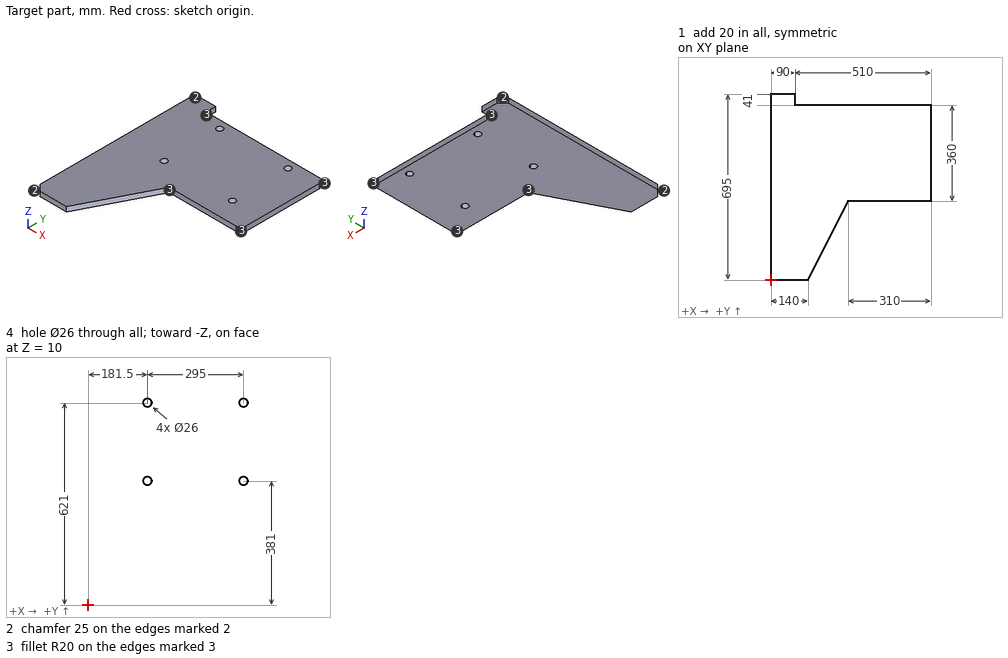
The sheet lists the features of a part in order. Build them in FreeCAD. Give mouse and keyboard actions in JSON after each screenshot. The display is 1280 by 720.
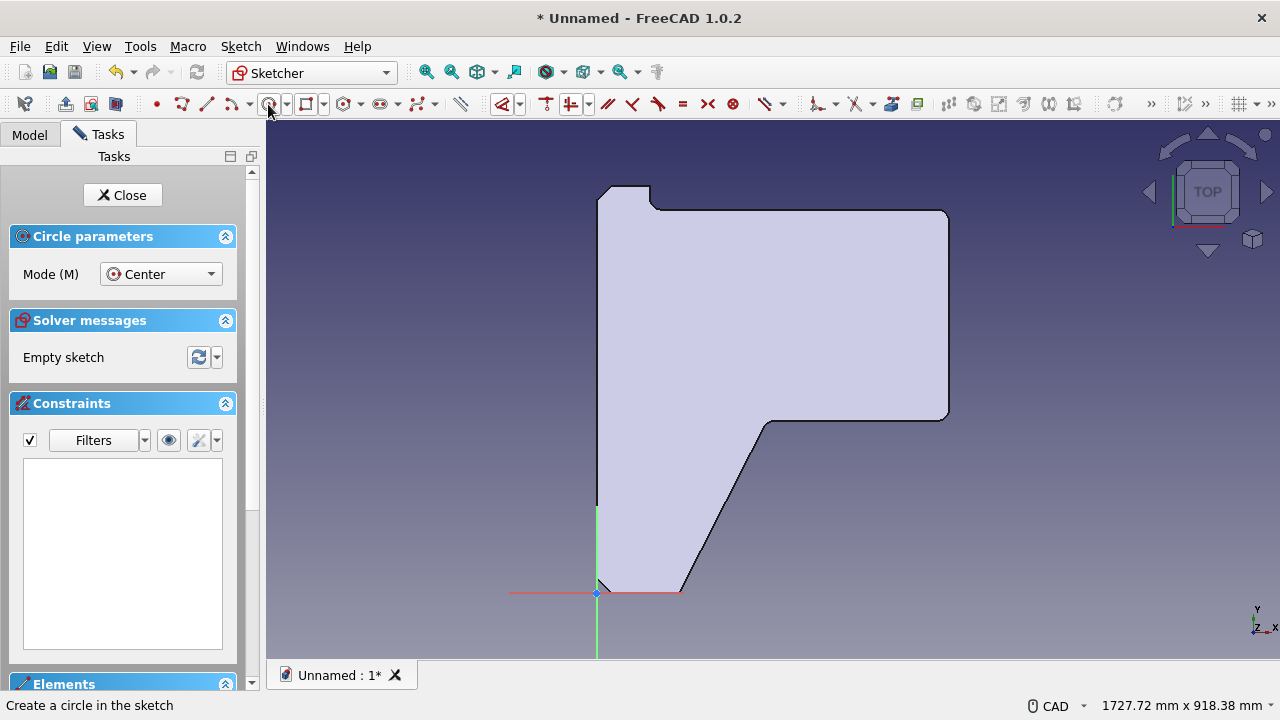
{"action": "scroll", "coordinate": [703, 229], "scroll_direction": "up", "scroll_amount": 6}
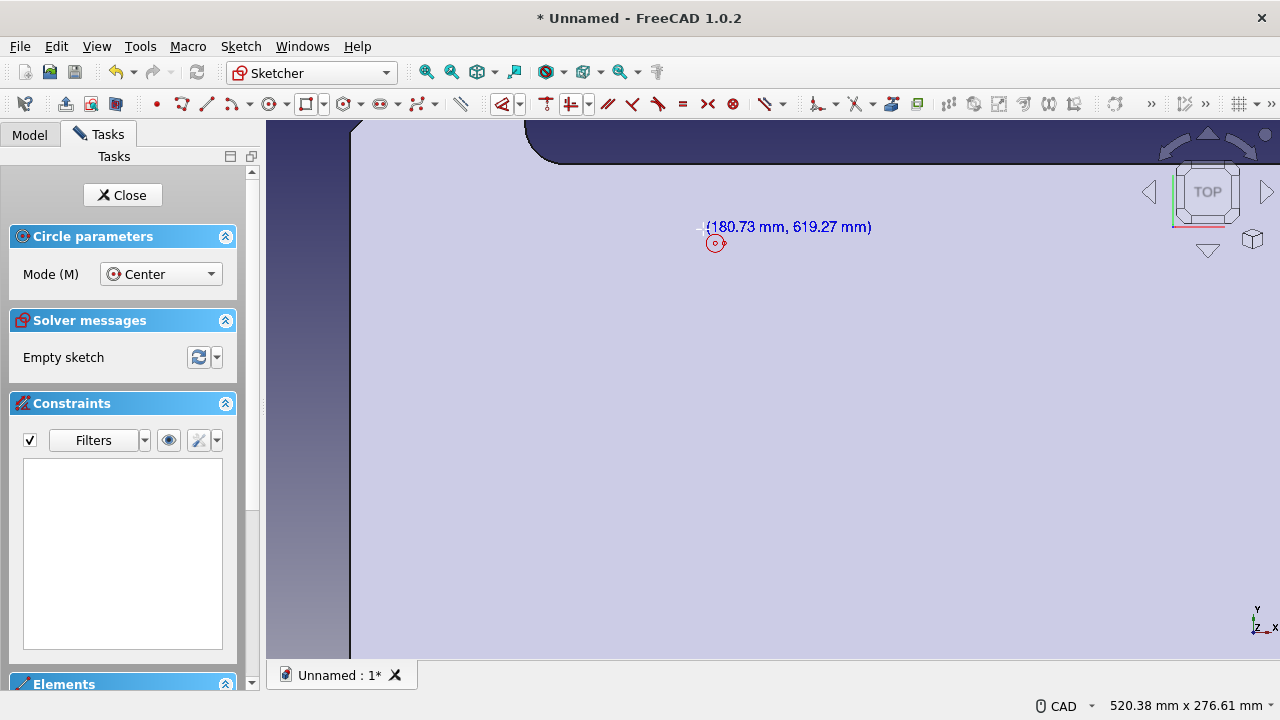
{"action": "left_click", "coordinate": [704, 228]}
{"action": "left_click", "coordinate": [721, 211]}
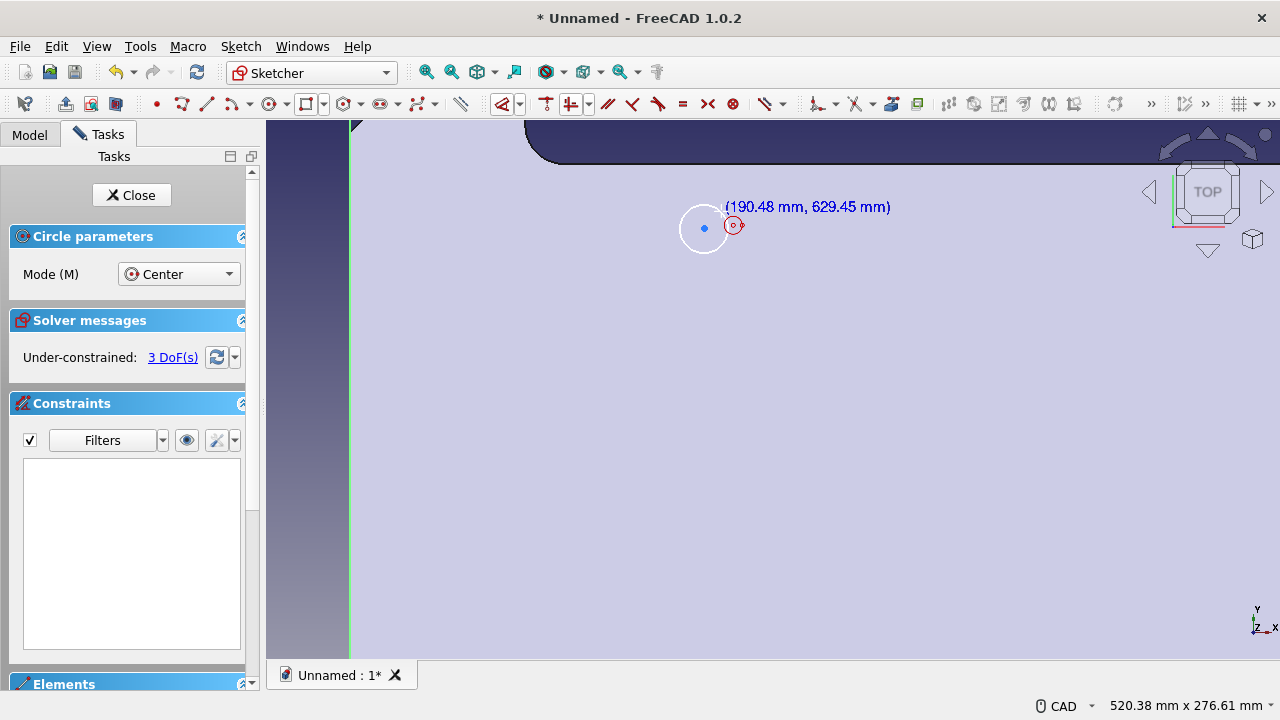
{"action": "scroll", "coordinate": [652, 204], "scroll_direction": "down", "scroll_amount": 6}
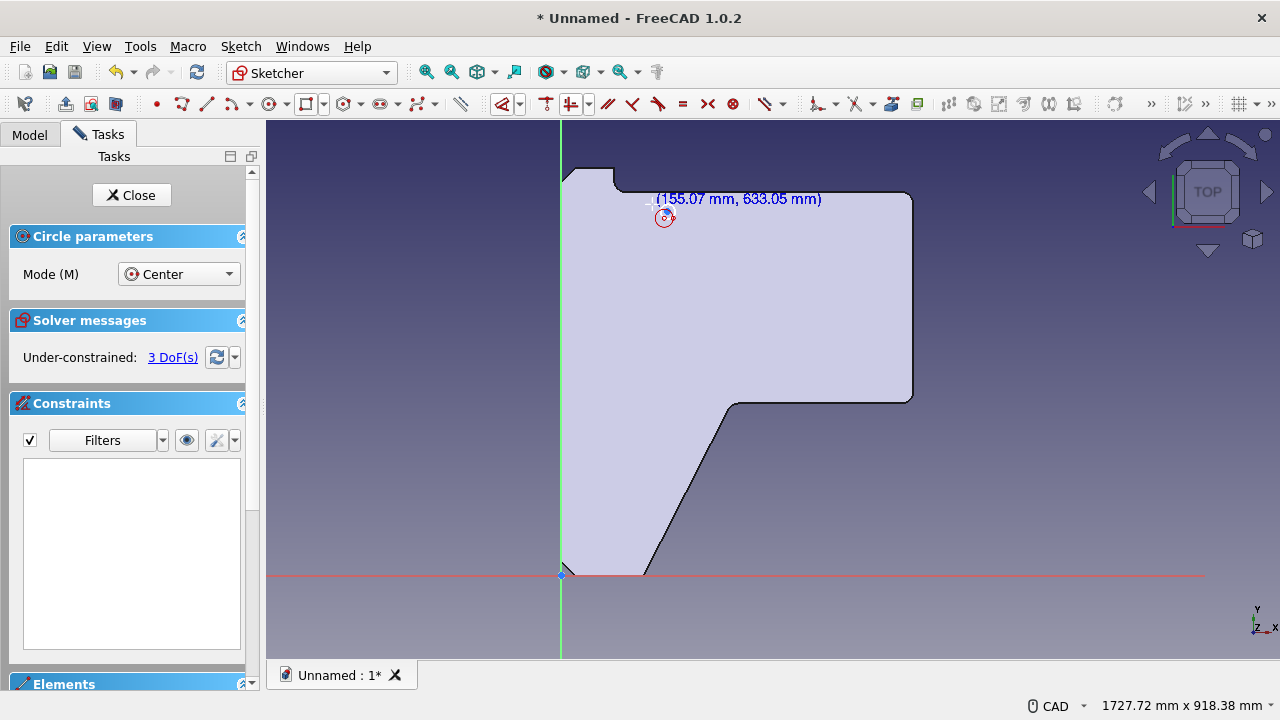
{"action": "scroll", "coordinate": [841, 211], "scroll_direction": "up", "scroll_amount": 6}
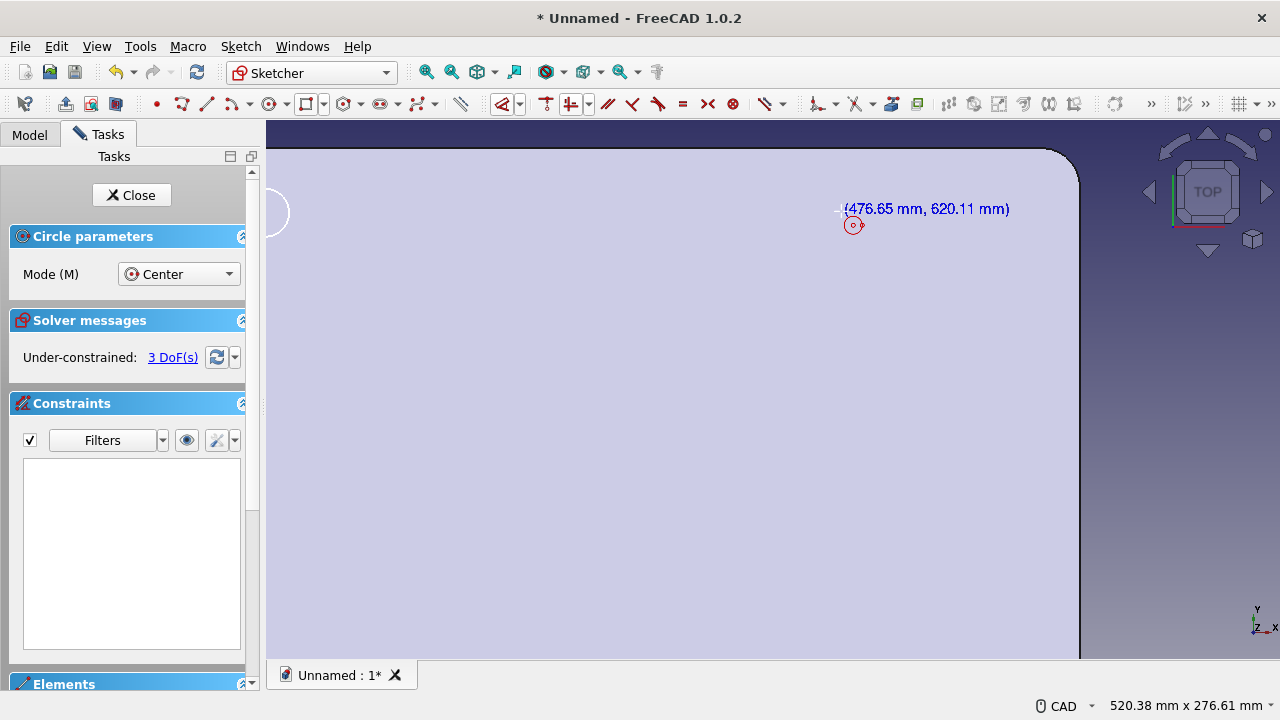
{"action": "left_click", "coordinate": [839, 212]}
{"action": "left_click", "coordinate": [857, 194]}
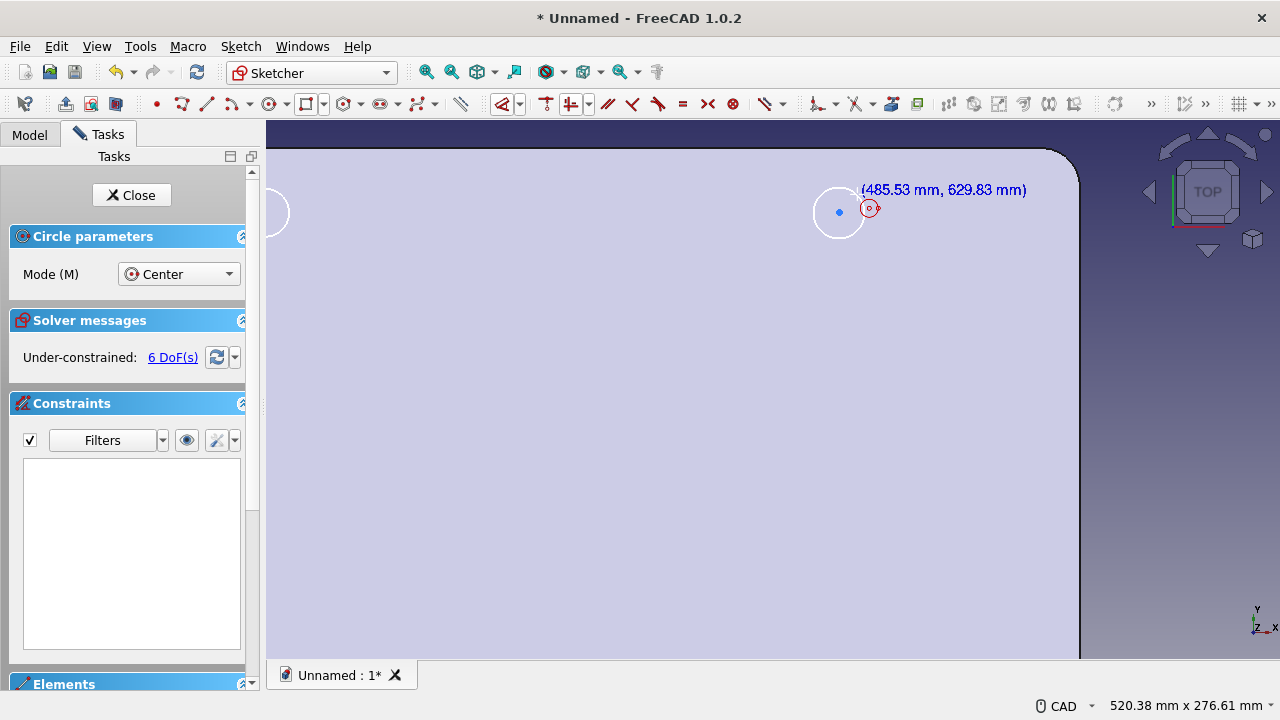
{"action": "scroll", "coordinate": [841, 211], "scroll_direction": "down", "scroll_amount": 6}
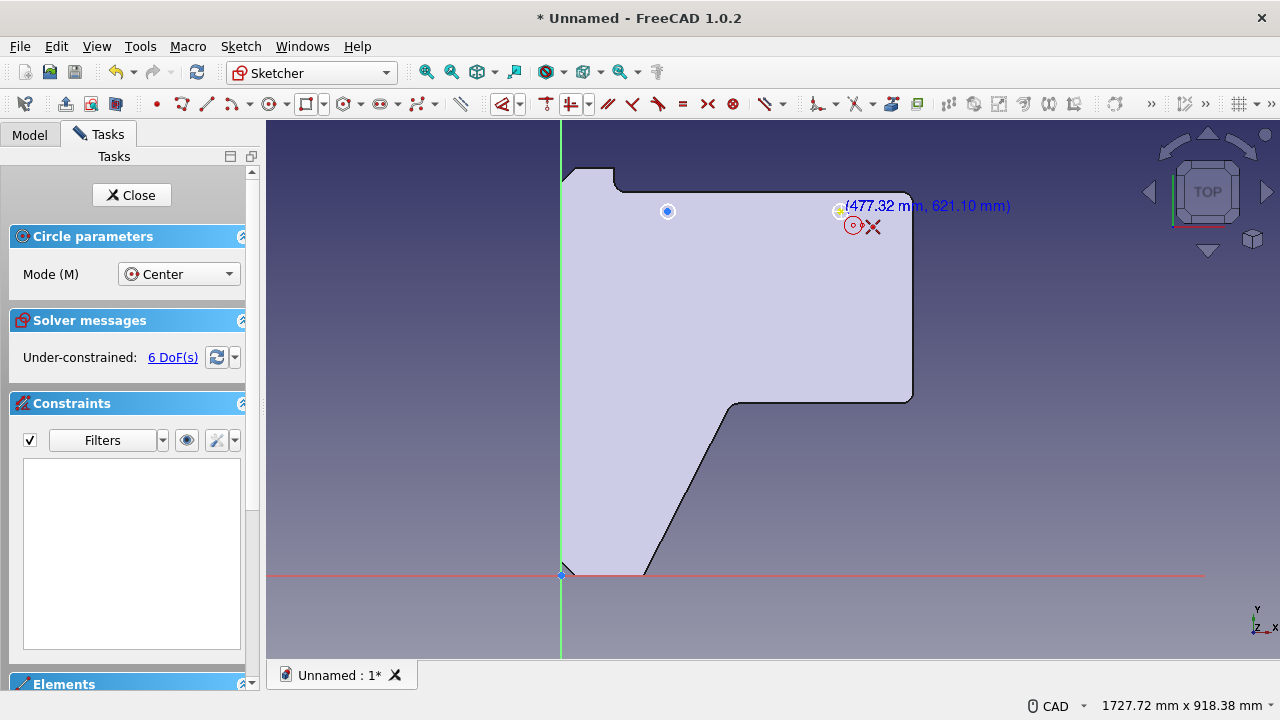
{"action": "scroll", "coordinate": [841, 352], "scroll_direction": "up", "scroll_amount": 6}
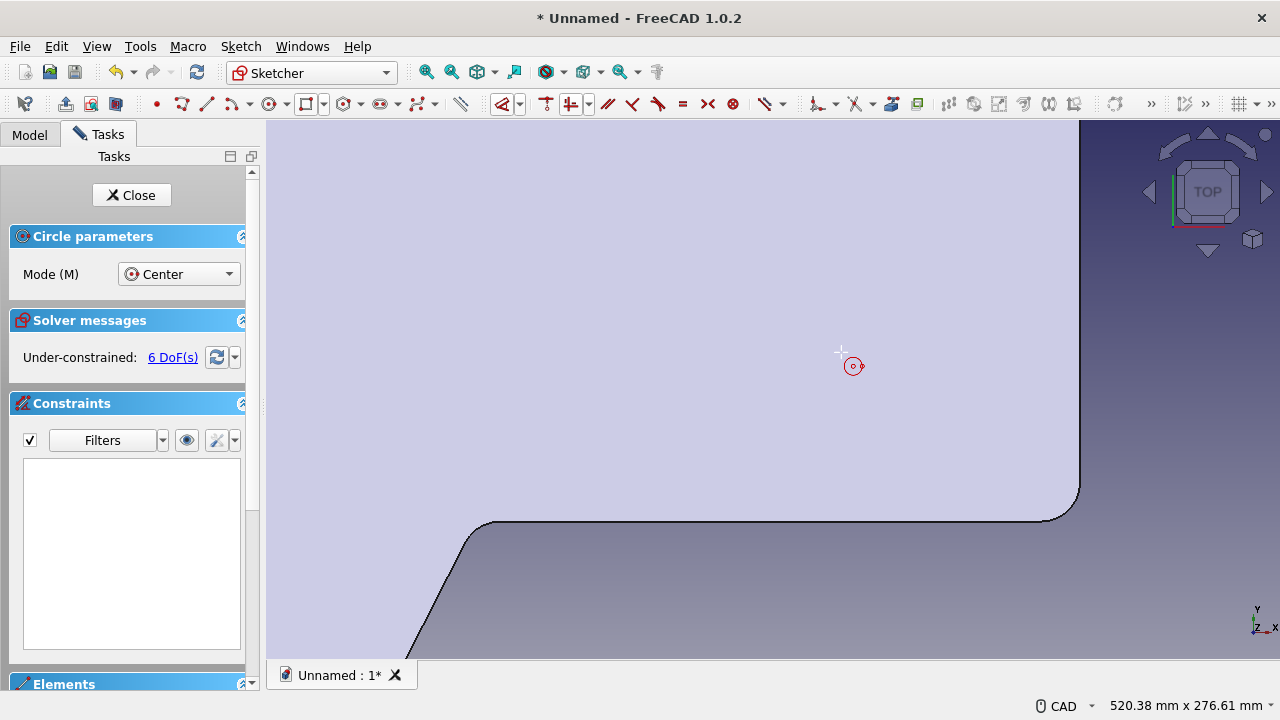
{"action": "left_click", "coordinate": [839, 352]}
{"action": "left_click", "coordinate": [857, 334]}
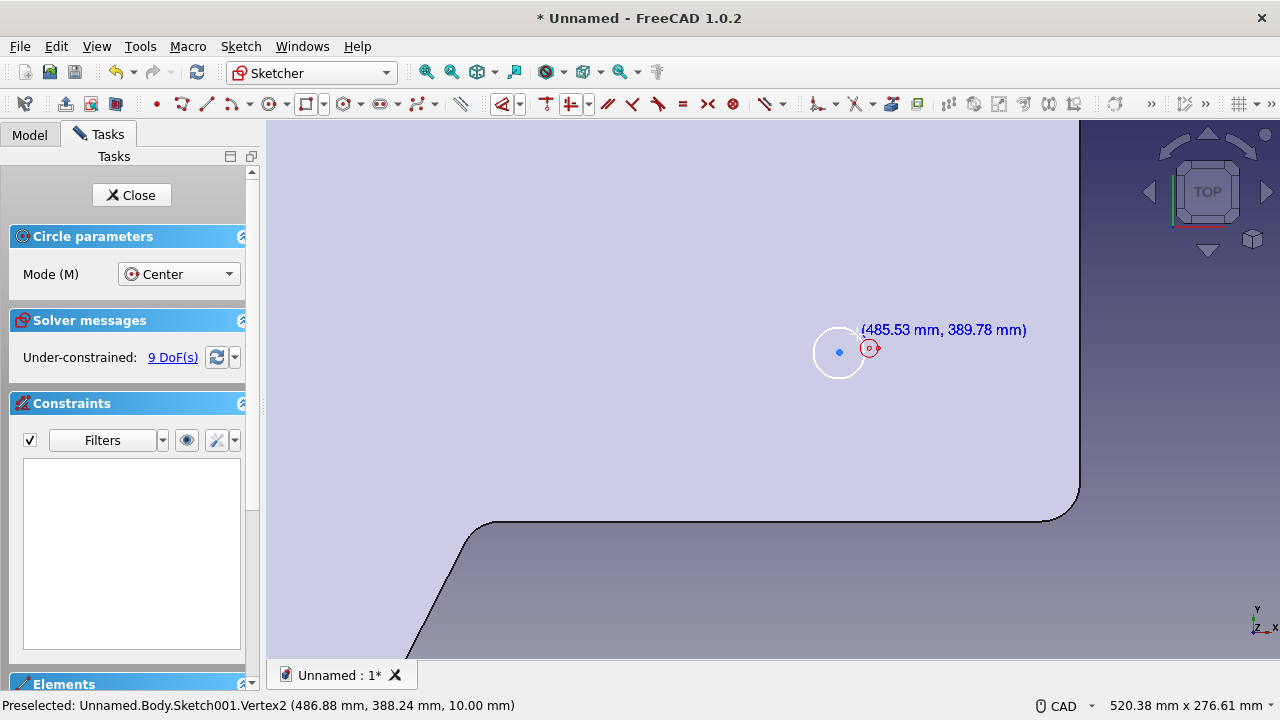
{"action": "scroll", "coordinate": [841, 352], "scroll_direction": "down", "scroll_amount": 6}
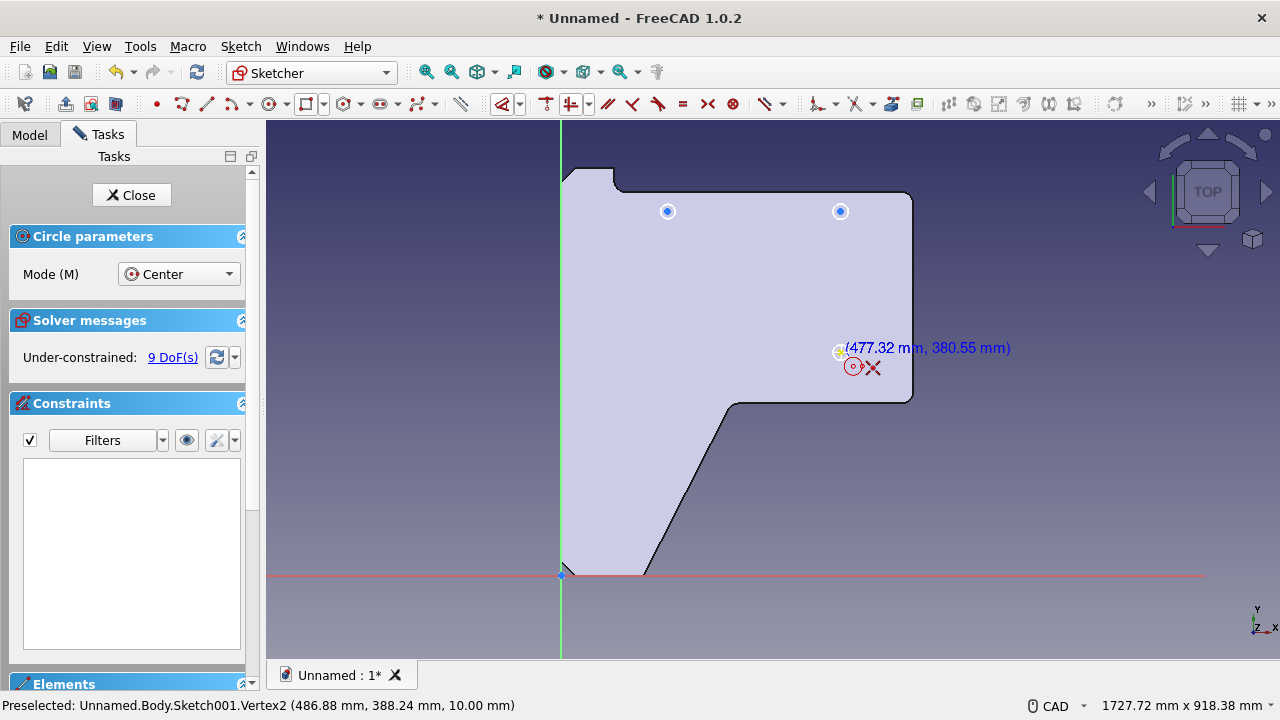
{"action": "scroll", "coordinate": [668, 352], "scroll_direction": "up", "scroll_amount": 6}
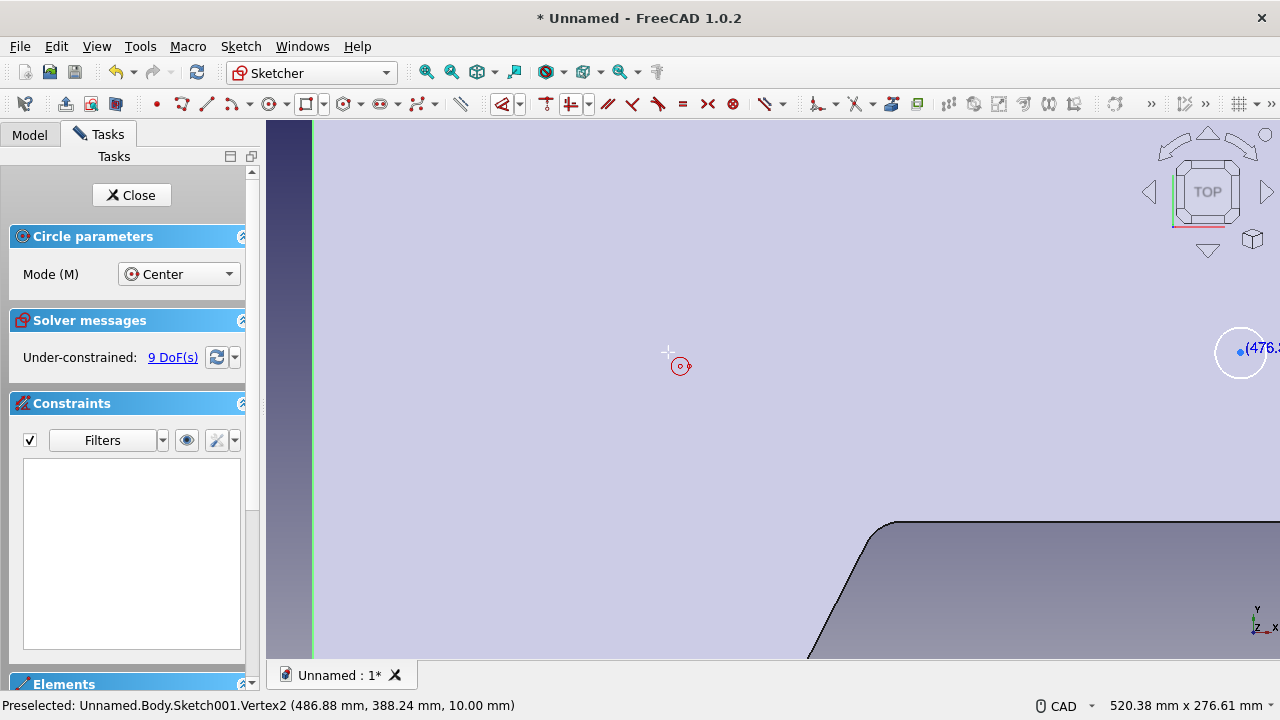
{"action": "left_click", "coordinate": [666, 352]}
{"action": "left_click", "coordinate": [684, 334]}
{"action": "key", "text": "Escape"}